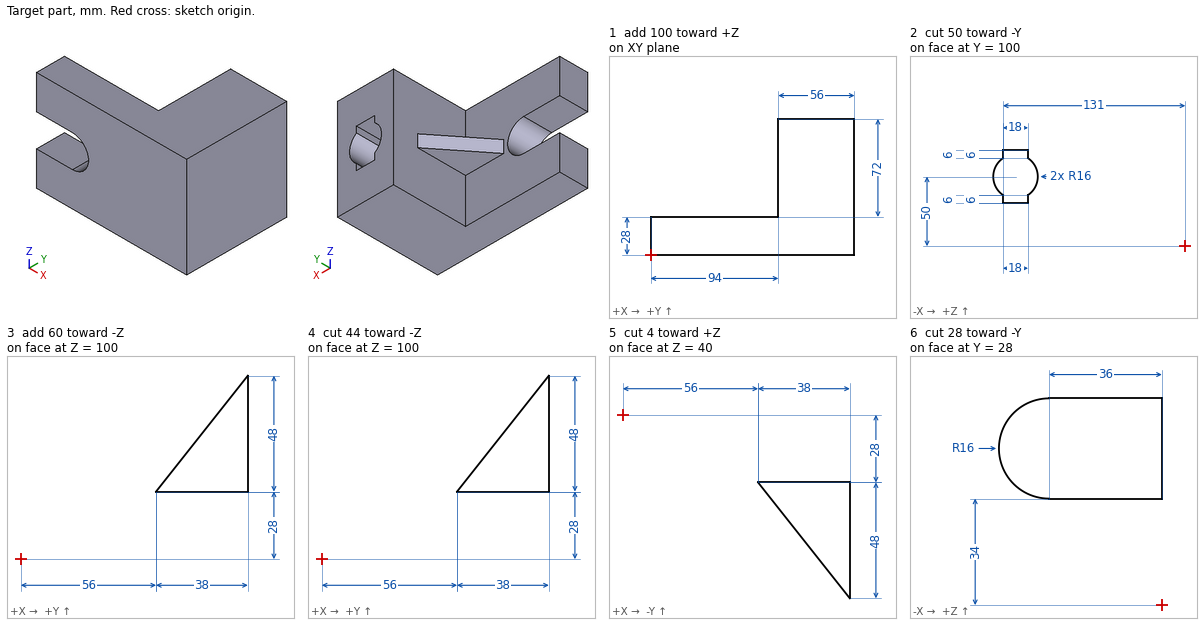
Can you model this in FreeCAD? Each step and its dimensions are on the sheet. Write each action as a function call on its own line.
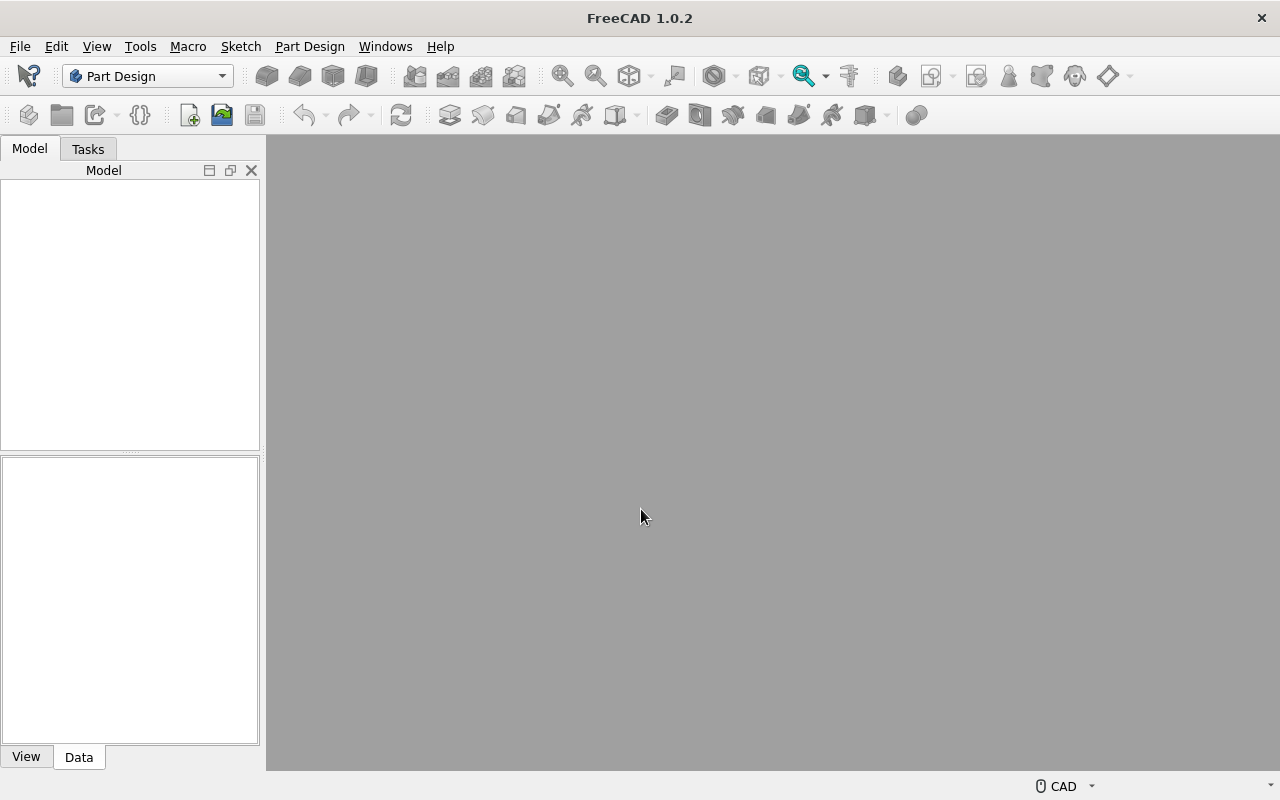
click(189, 116)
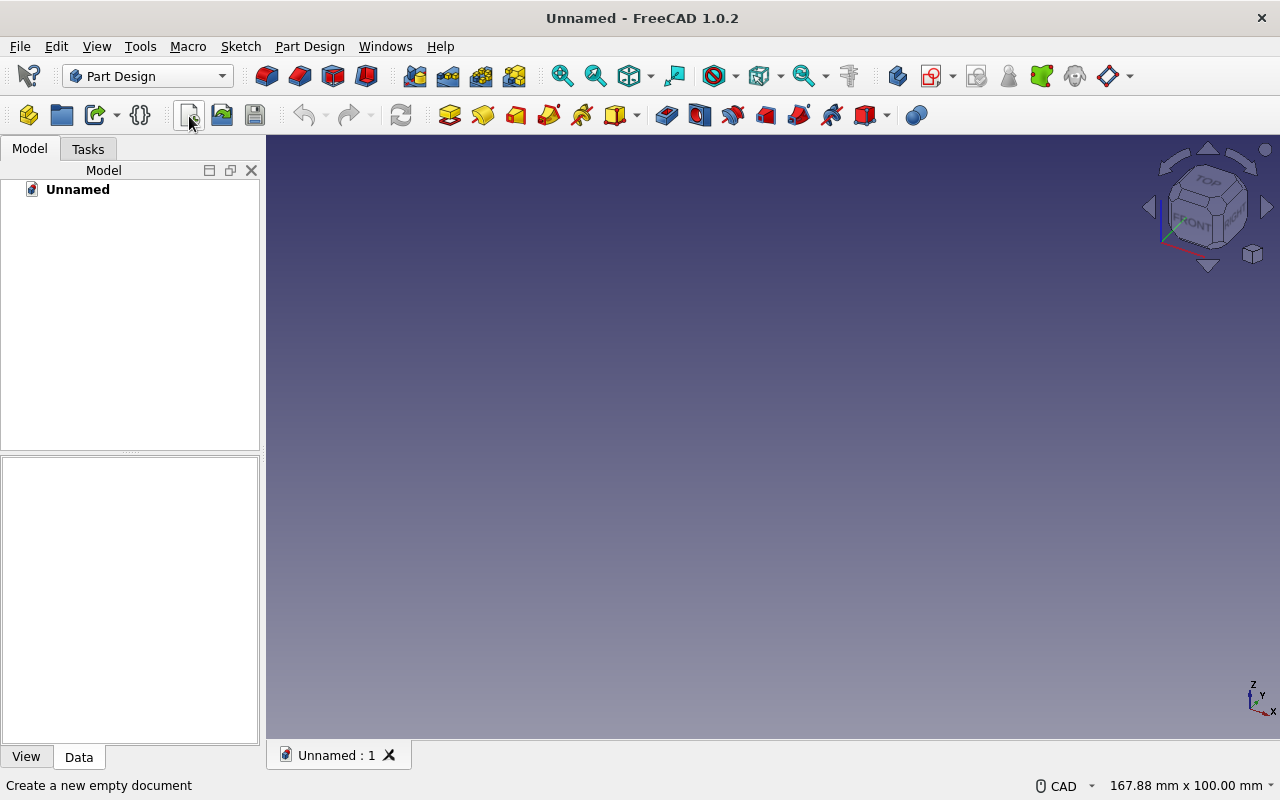
click(930, 76)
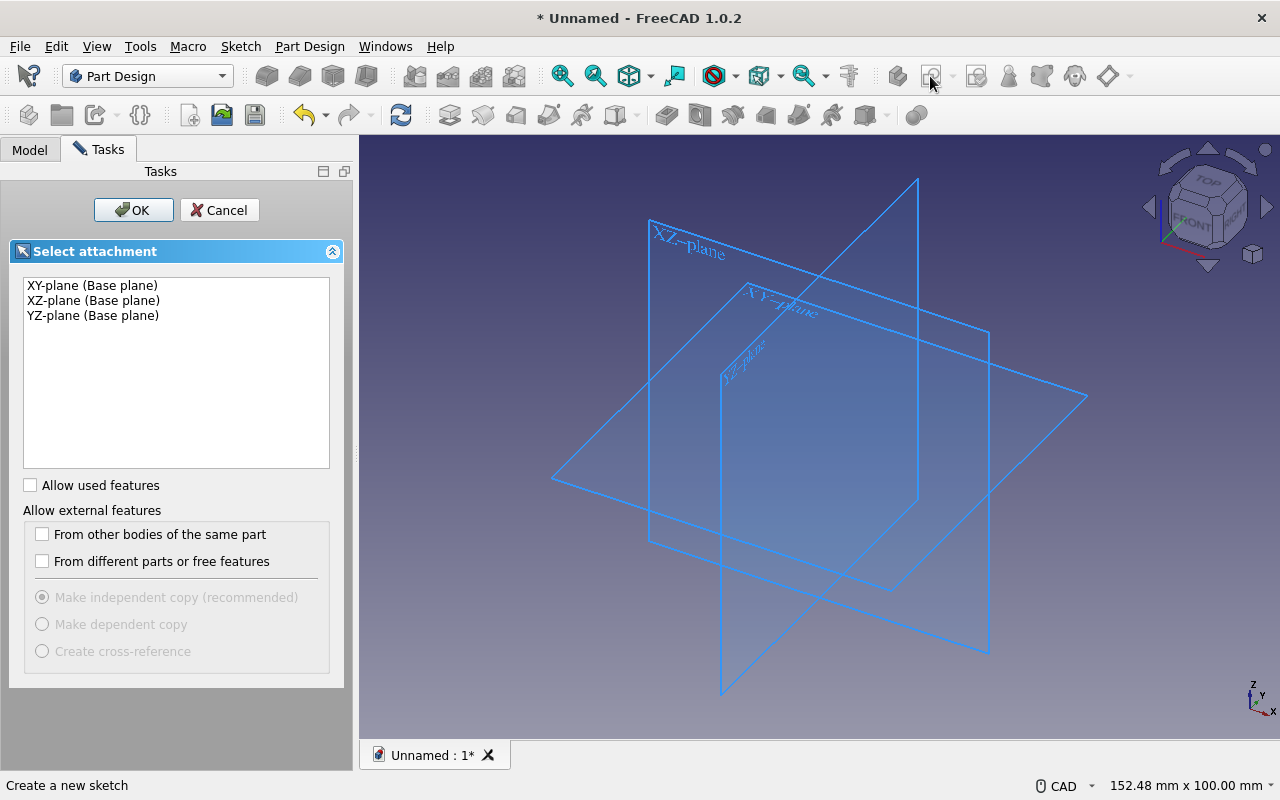
click(84, 286)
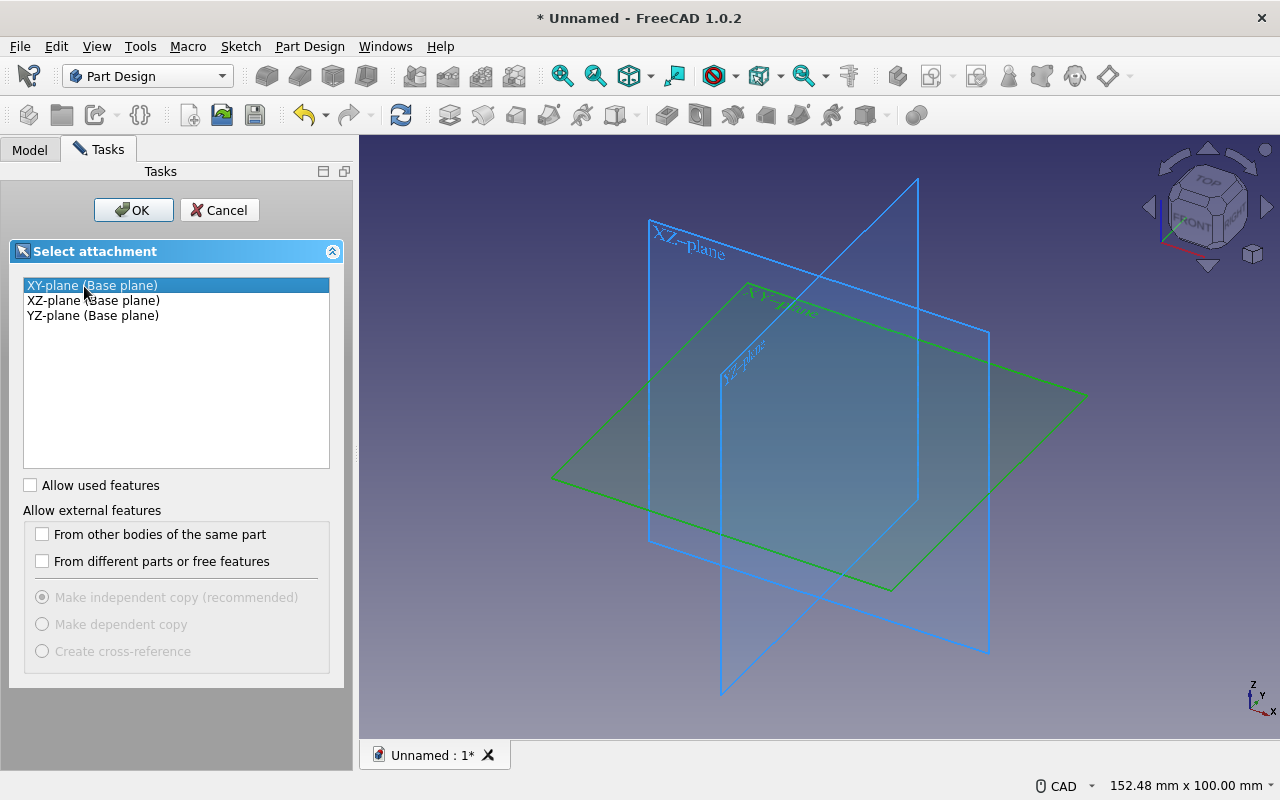
click(134, 210)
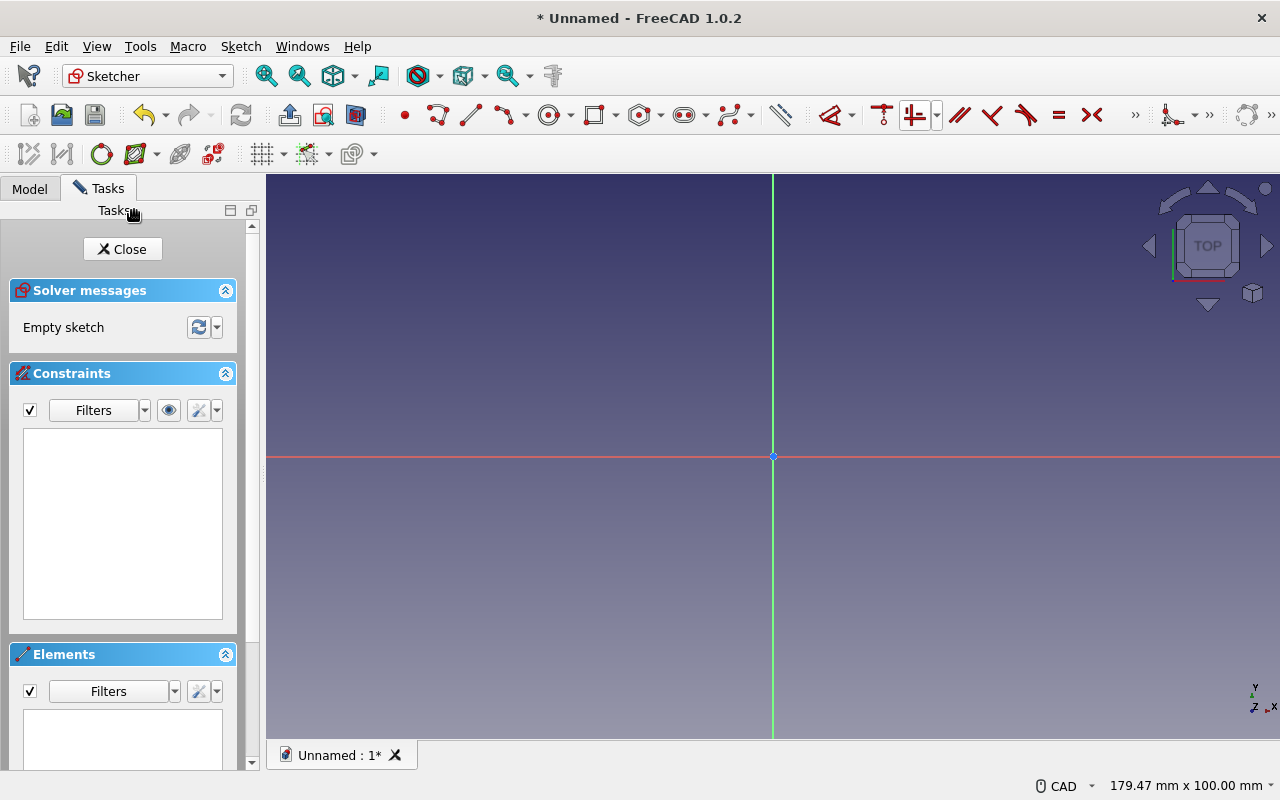
scroll(294, 711, down, 3)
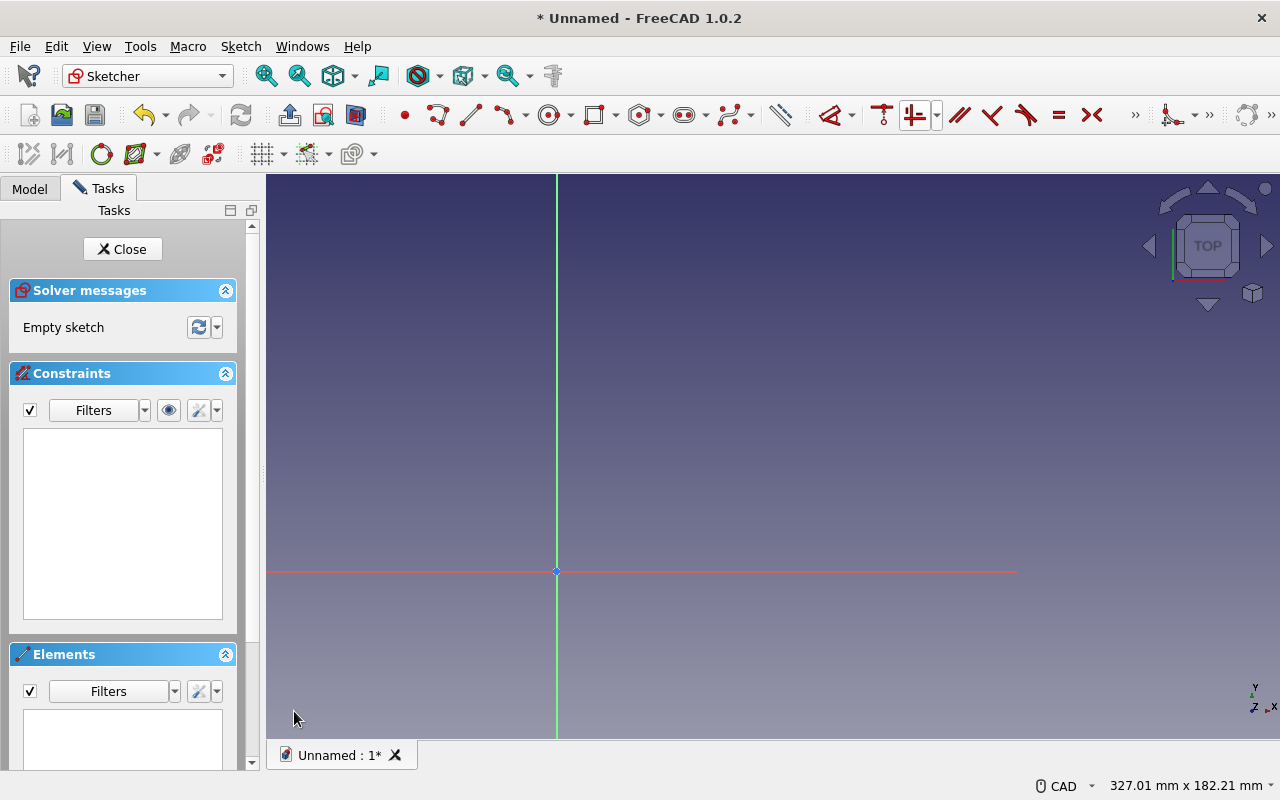
click(438, 116)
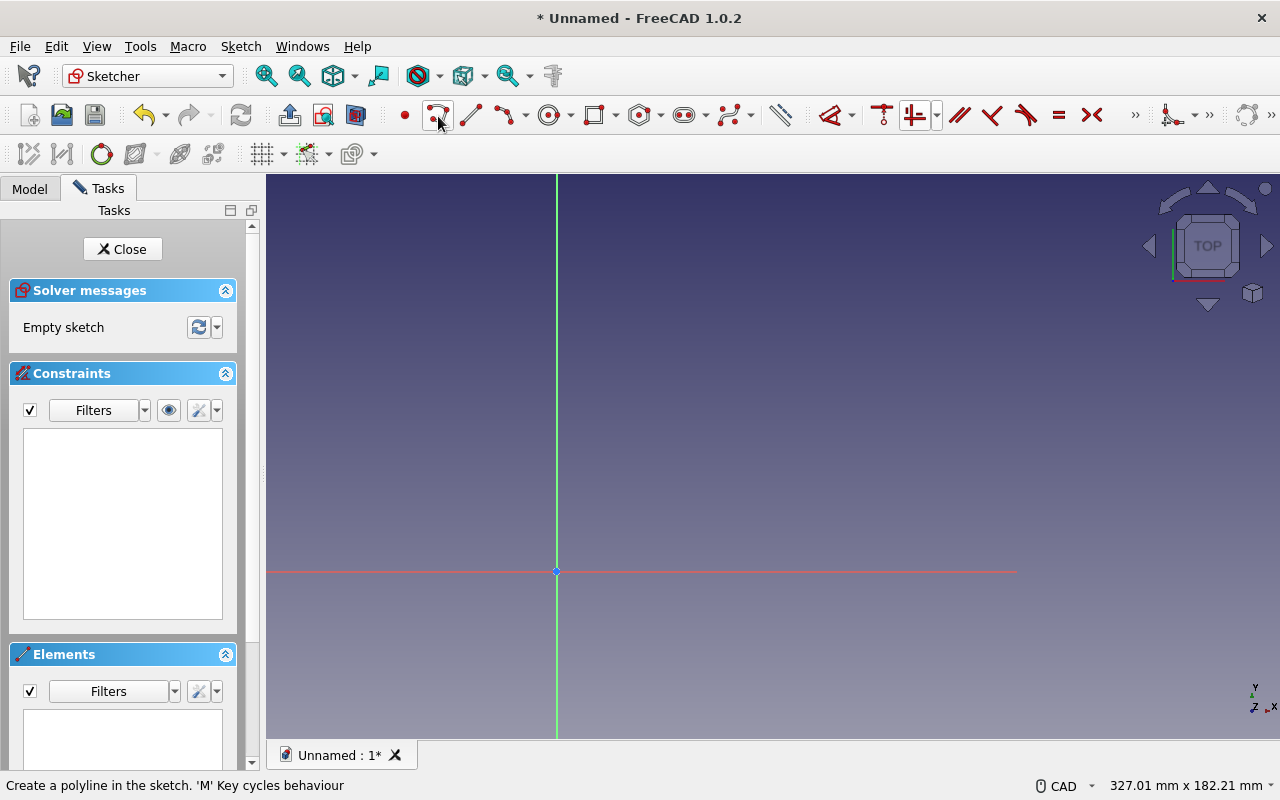
click(557, 572)
click(1022, 563)
click(1022, 262)
click(848, 262)
click(848, 485)
click(566, 485)
click(557, 572)
key(Escape)
key(Escape)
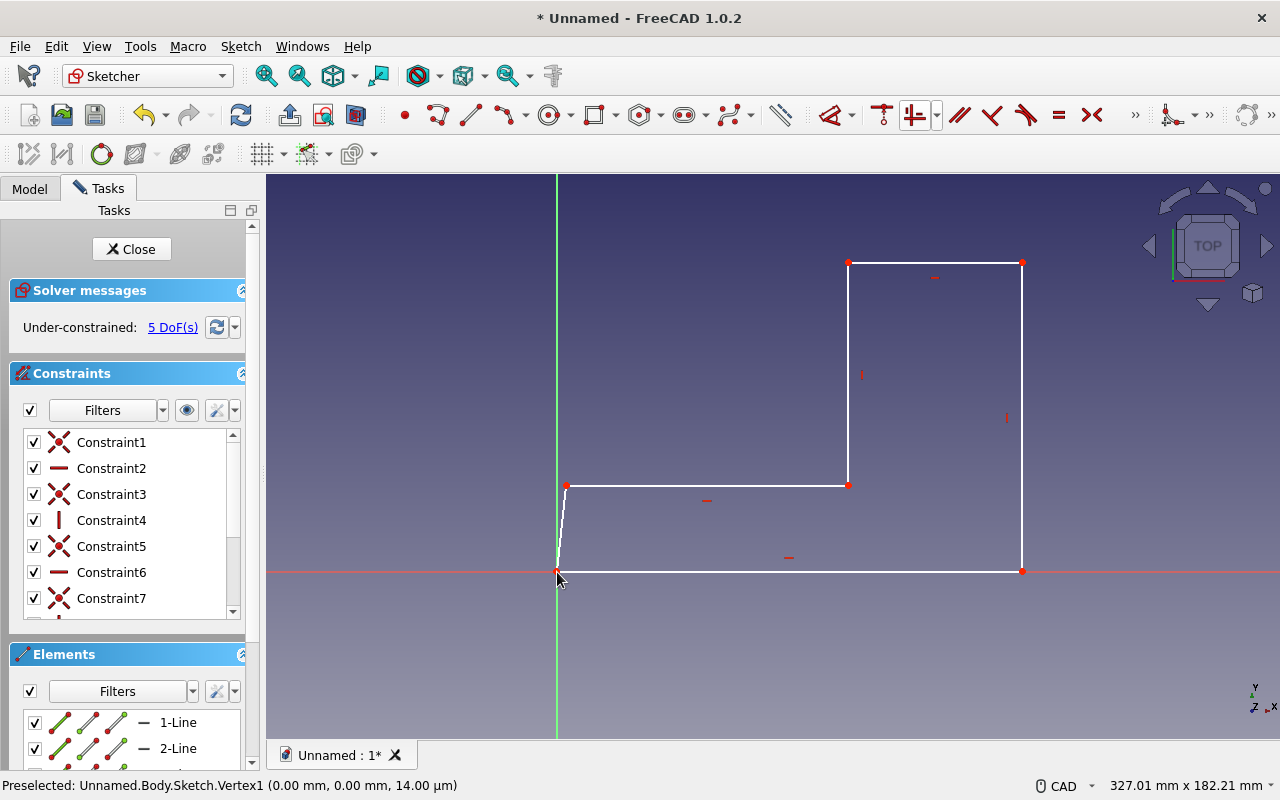
click(560, 546)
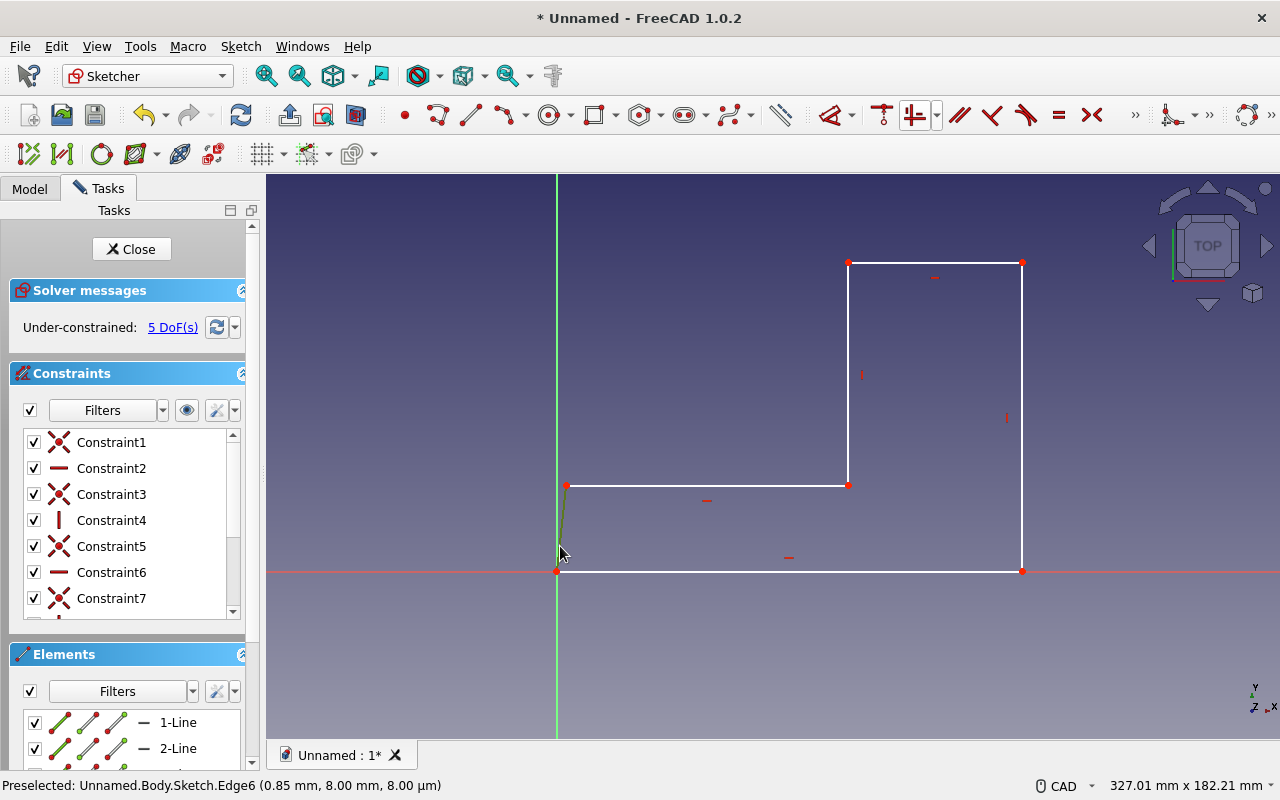
click(936, 116)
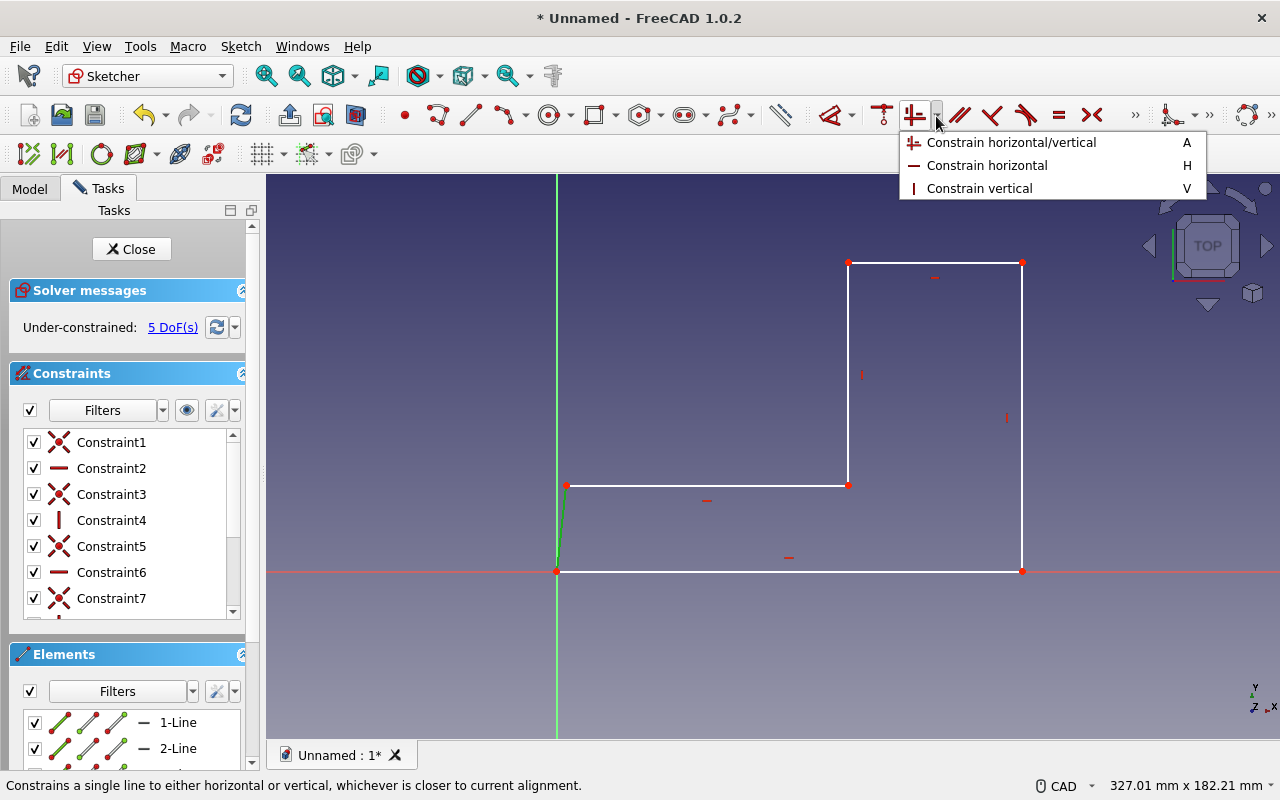
click(1053, 188)